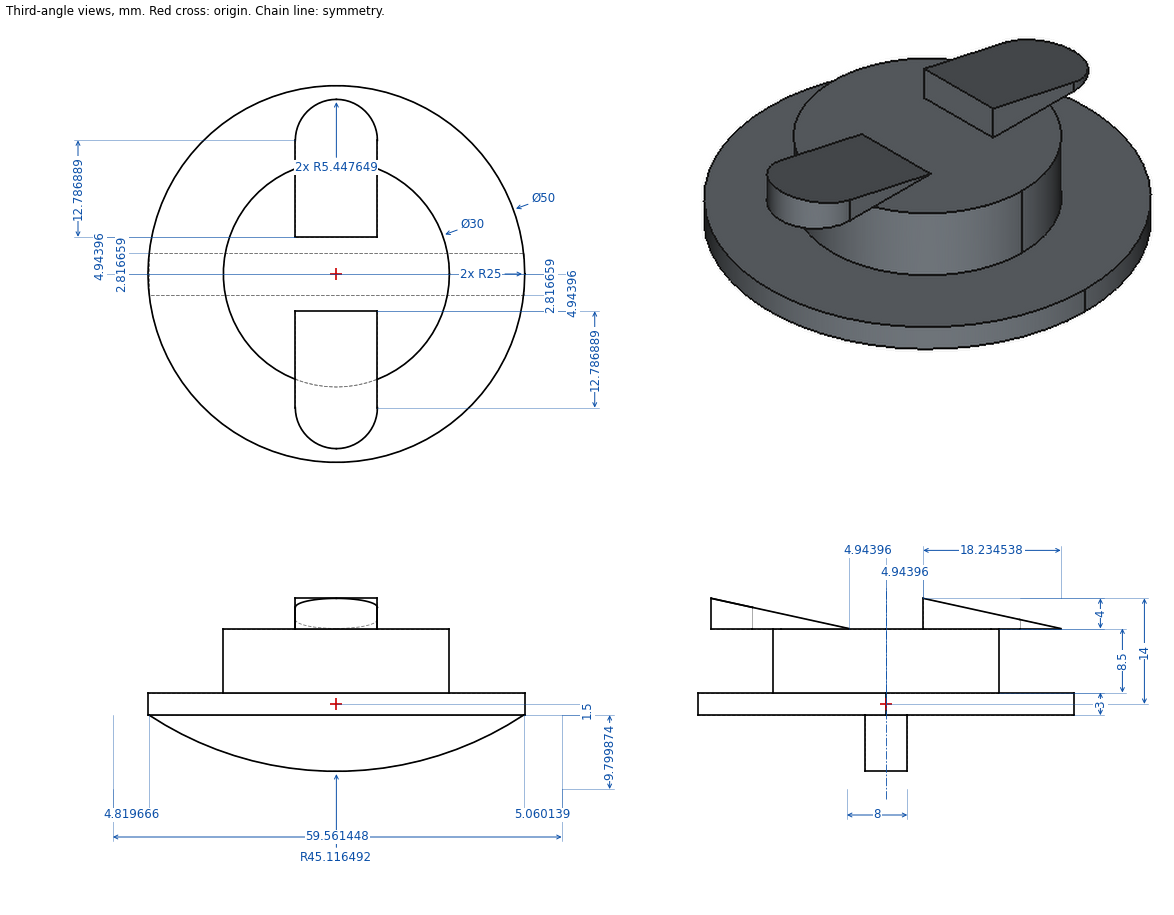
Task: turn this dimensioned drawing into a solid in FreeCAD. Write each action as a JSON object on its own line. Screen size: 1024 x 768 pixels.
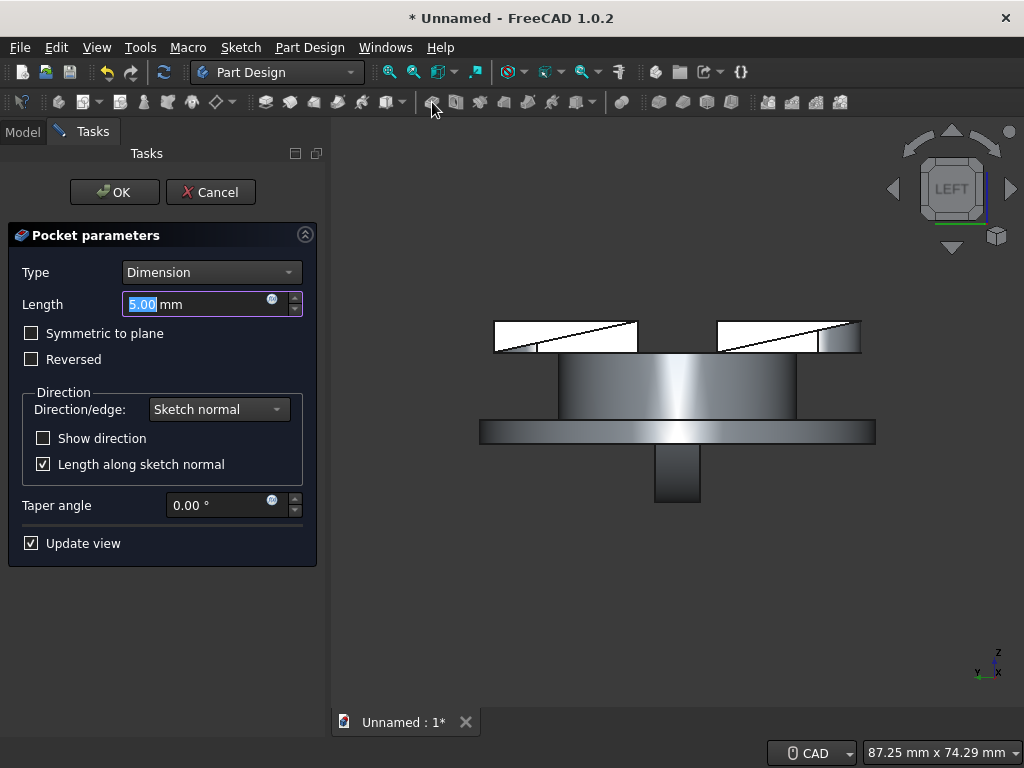
{"action": "left_click", "coordinate": [212, 272]}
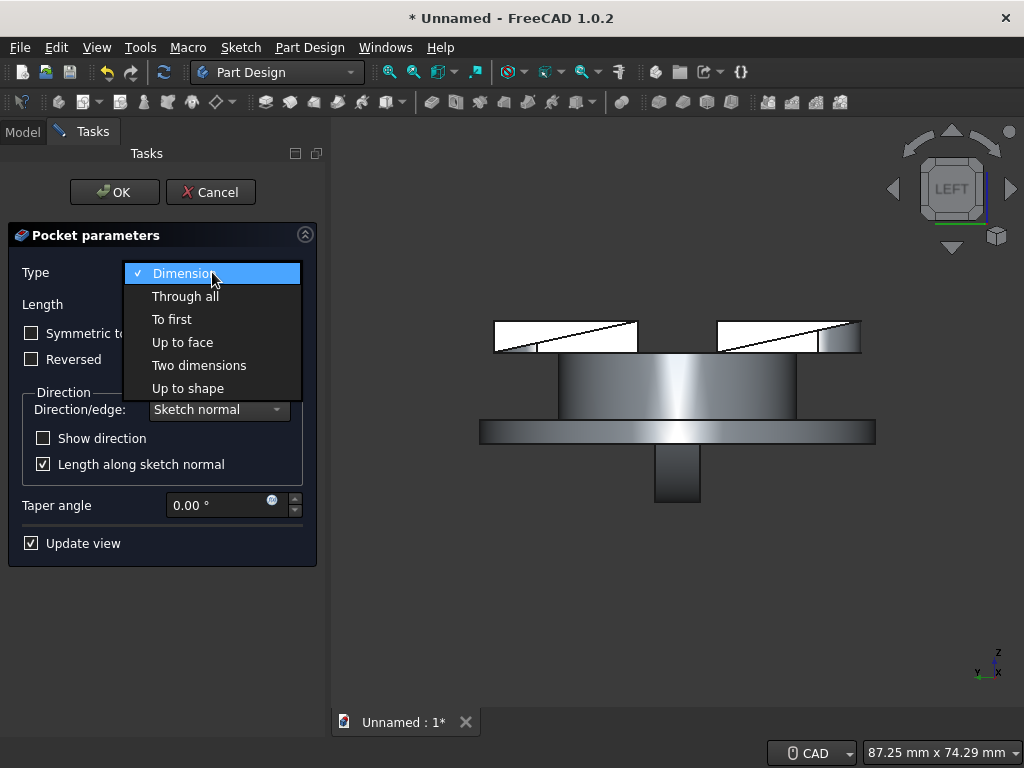
{"action": "left_click", "coordinate": [212, 296]}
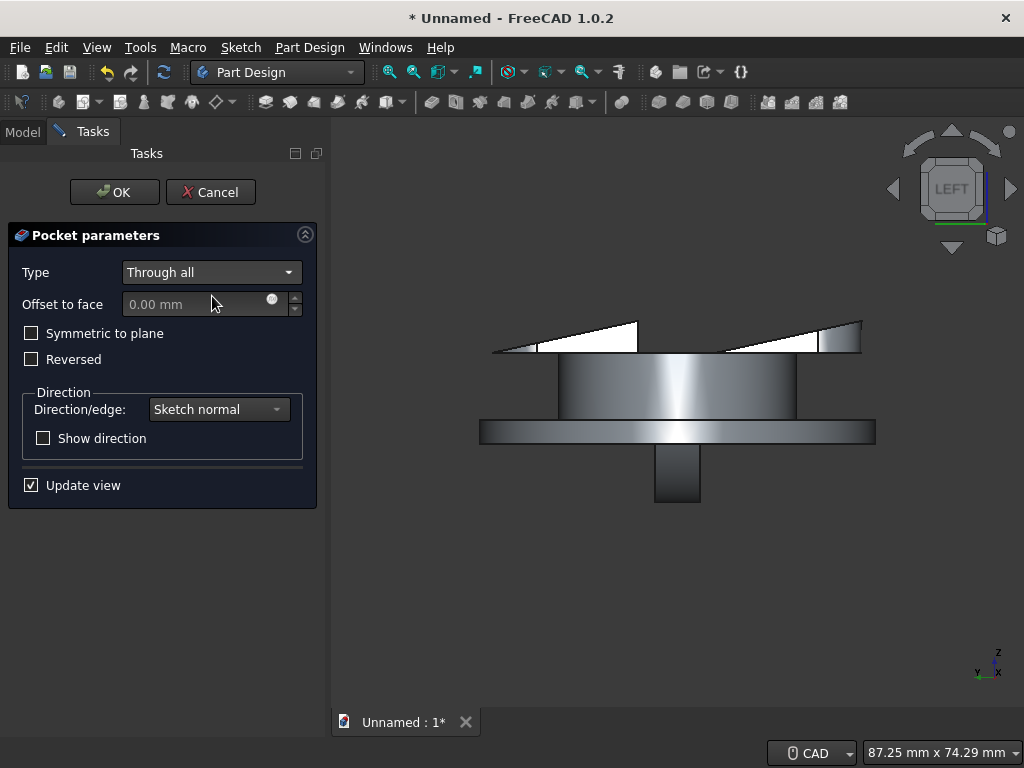
{"action": "left_click", "coordinate": [115, 192]}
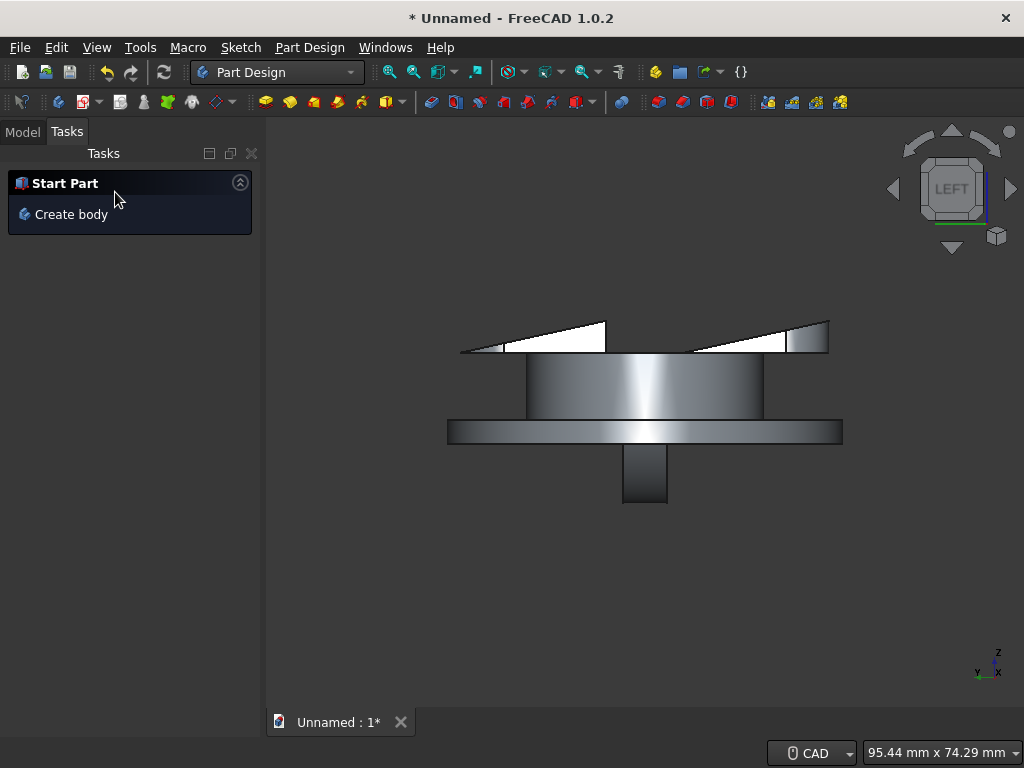
{"action": "key", "text": "0"}